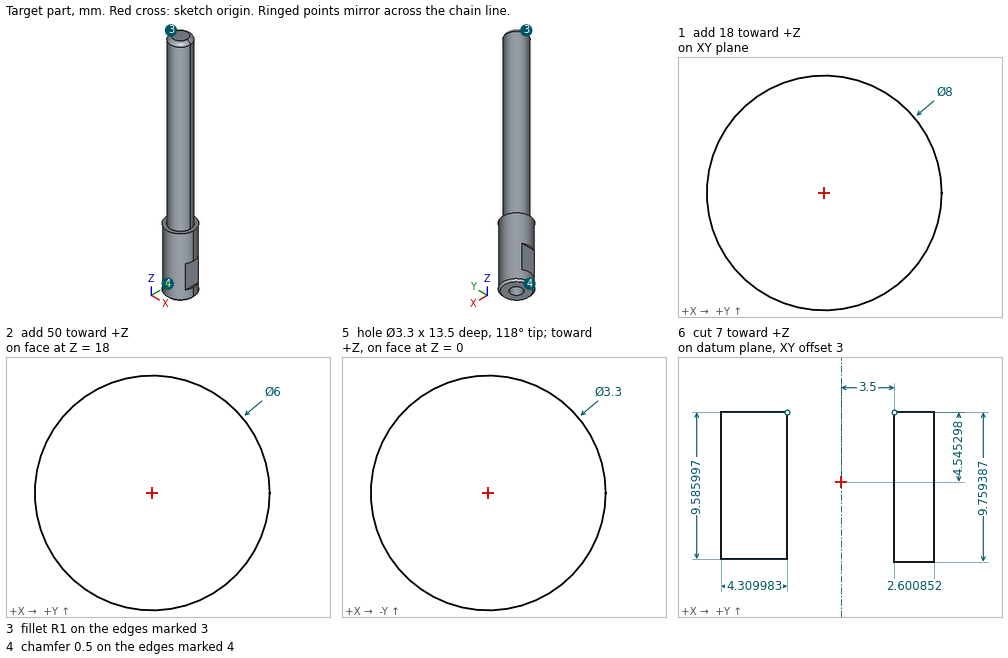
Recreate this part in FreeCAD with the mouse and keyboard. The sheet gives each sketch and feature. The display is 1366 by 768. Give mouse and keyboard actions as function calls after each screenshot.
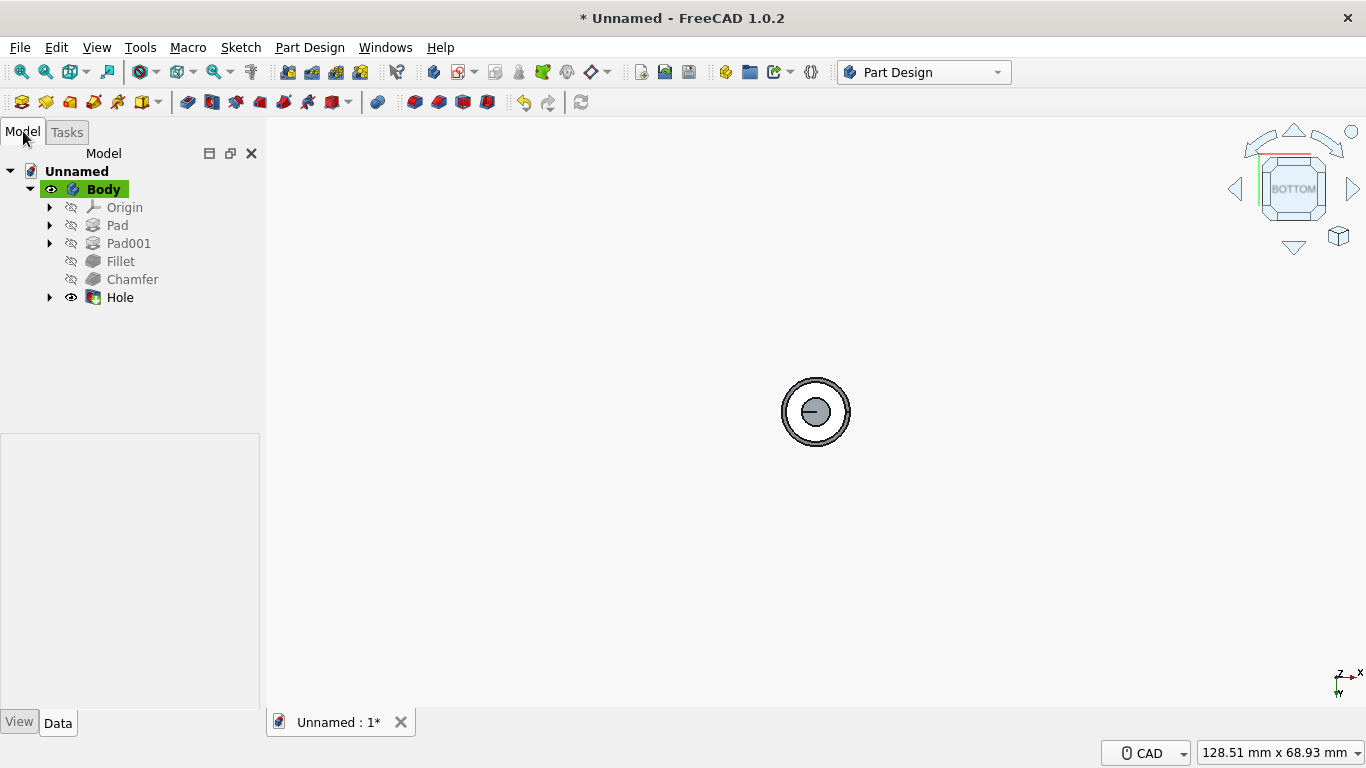
click(50, 207)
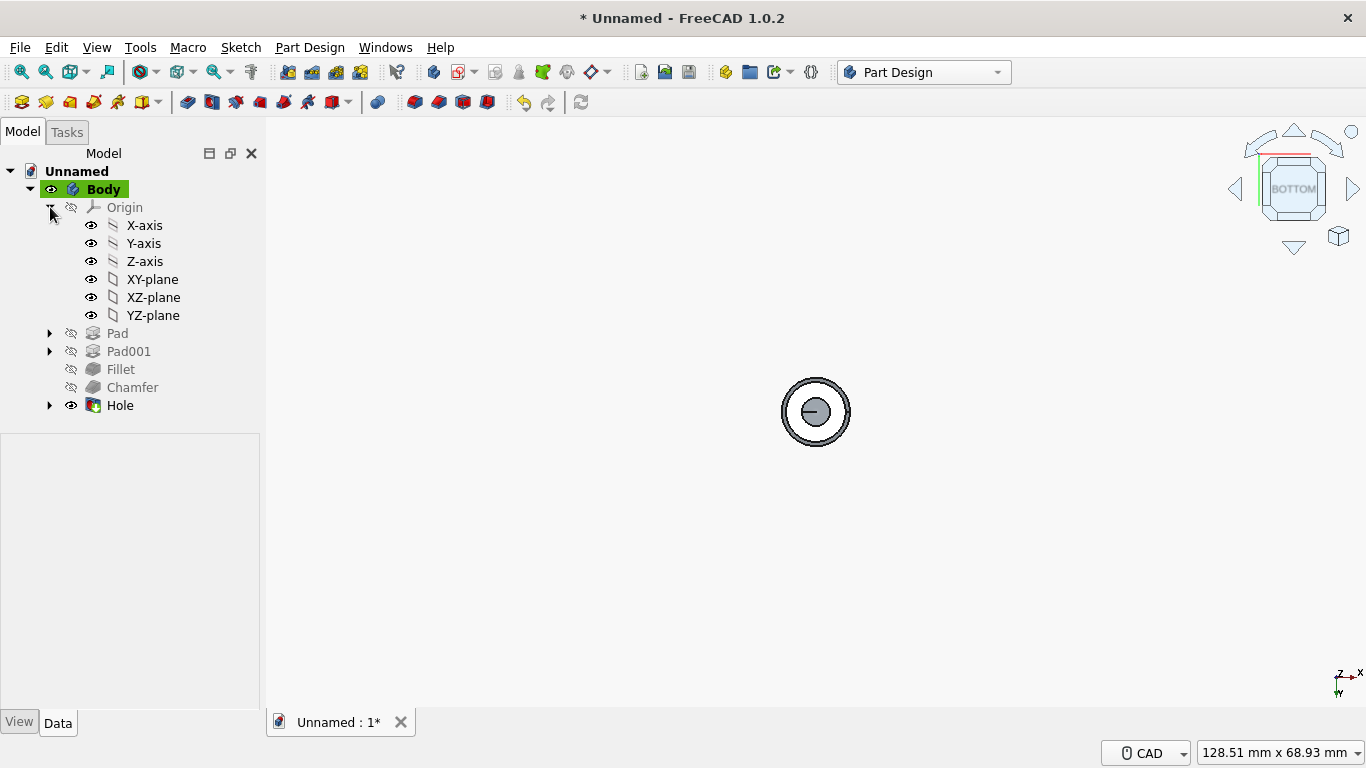
click(136, 279)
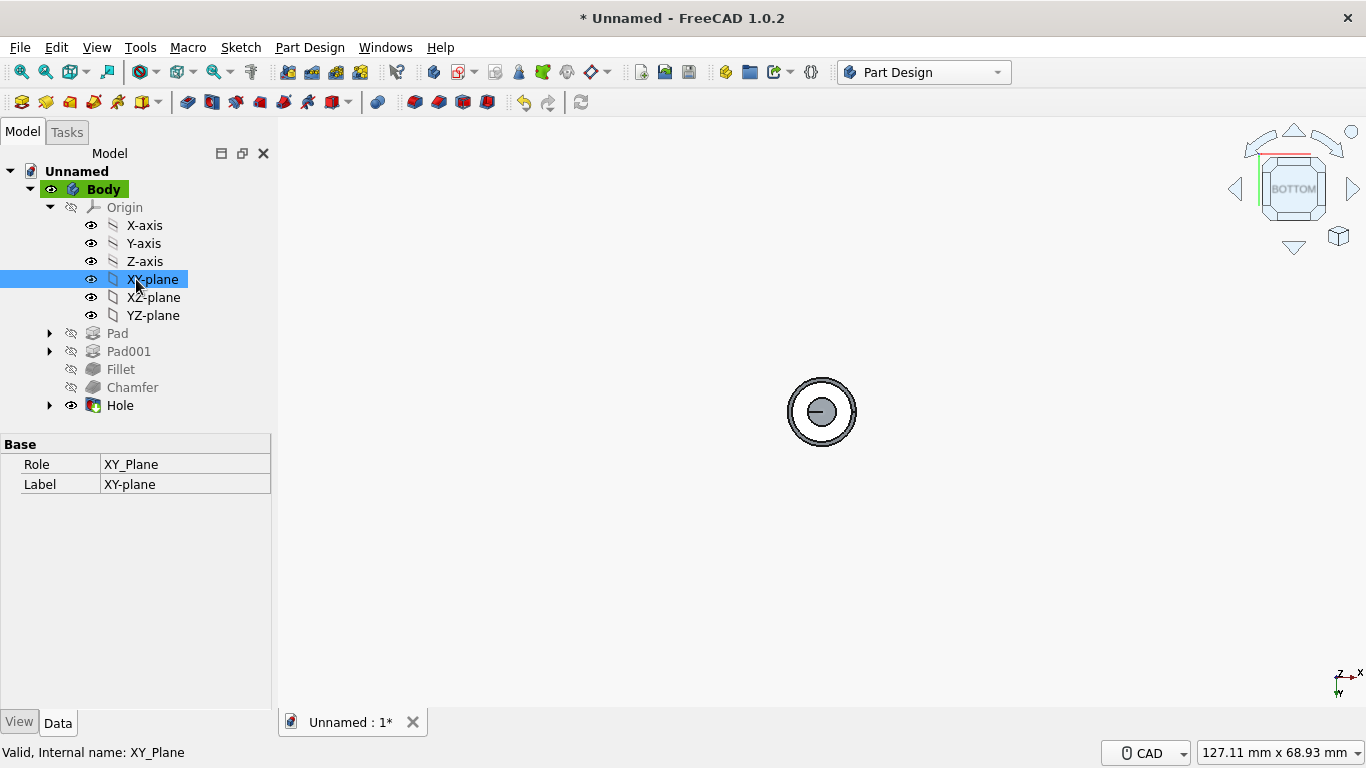
click(592, 72)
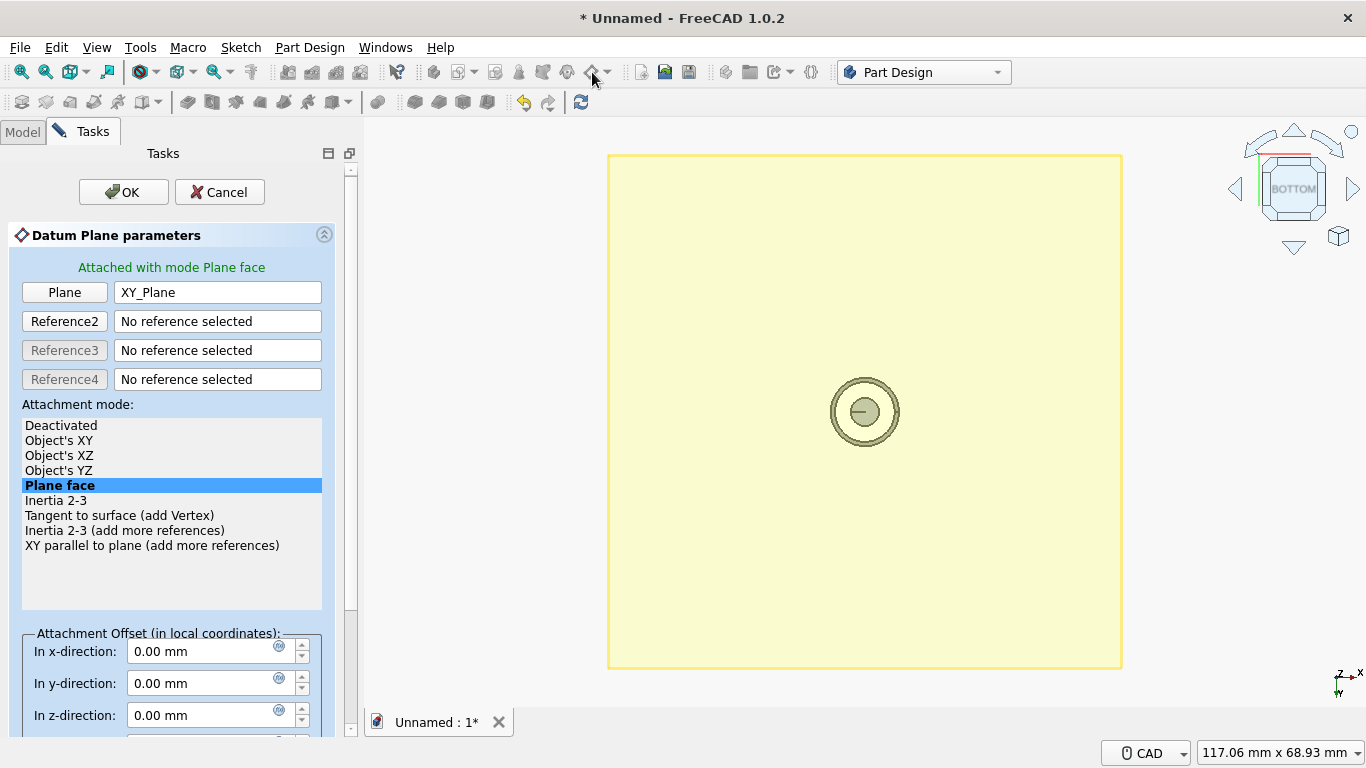
triple_click(210, 715)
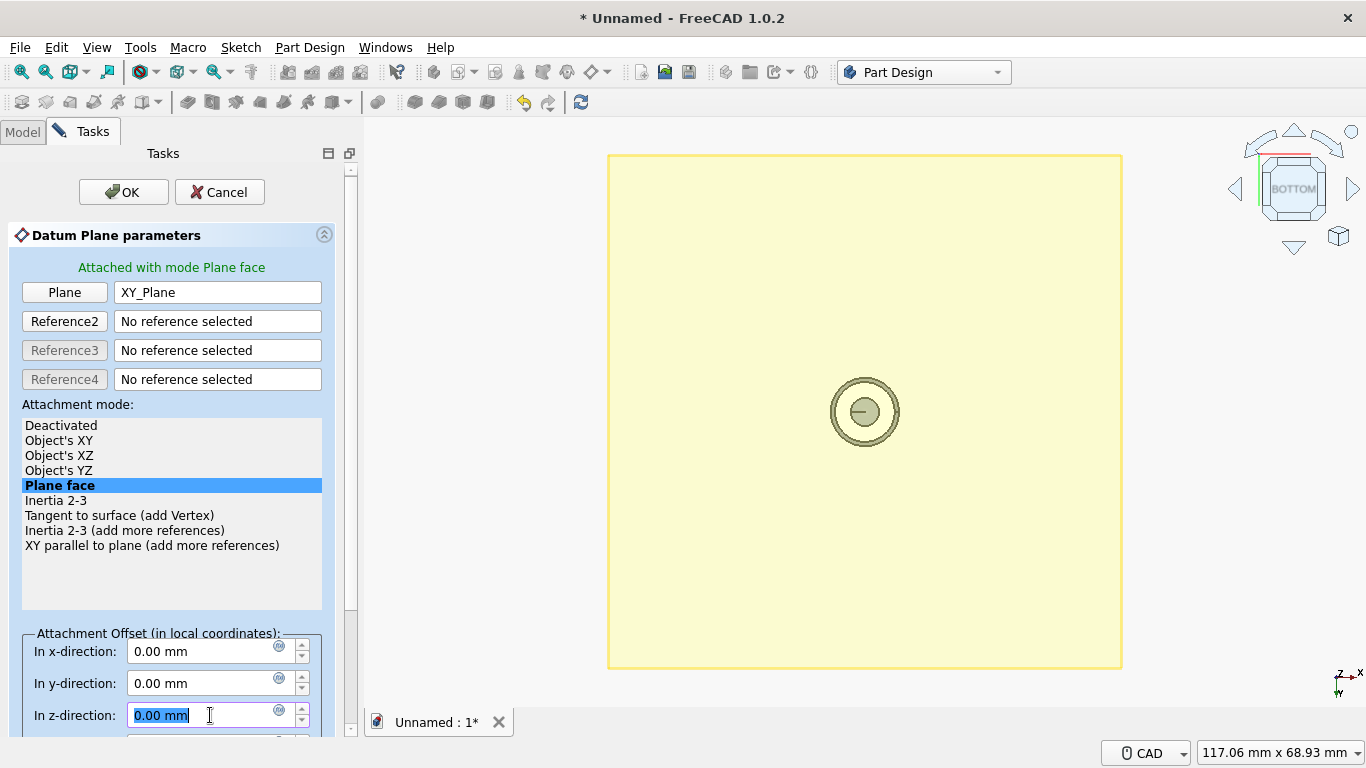
text(3)
key(Tab)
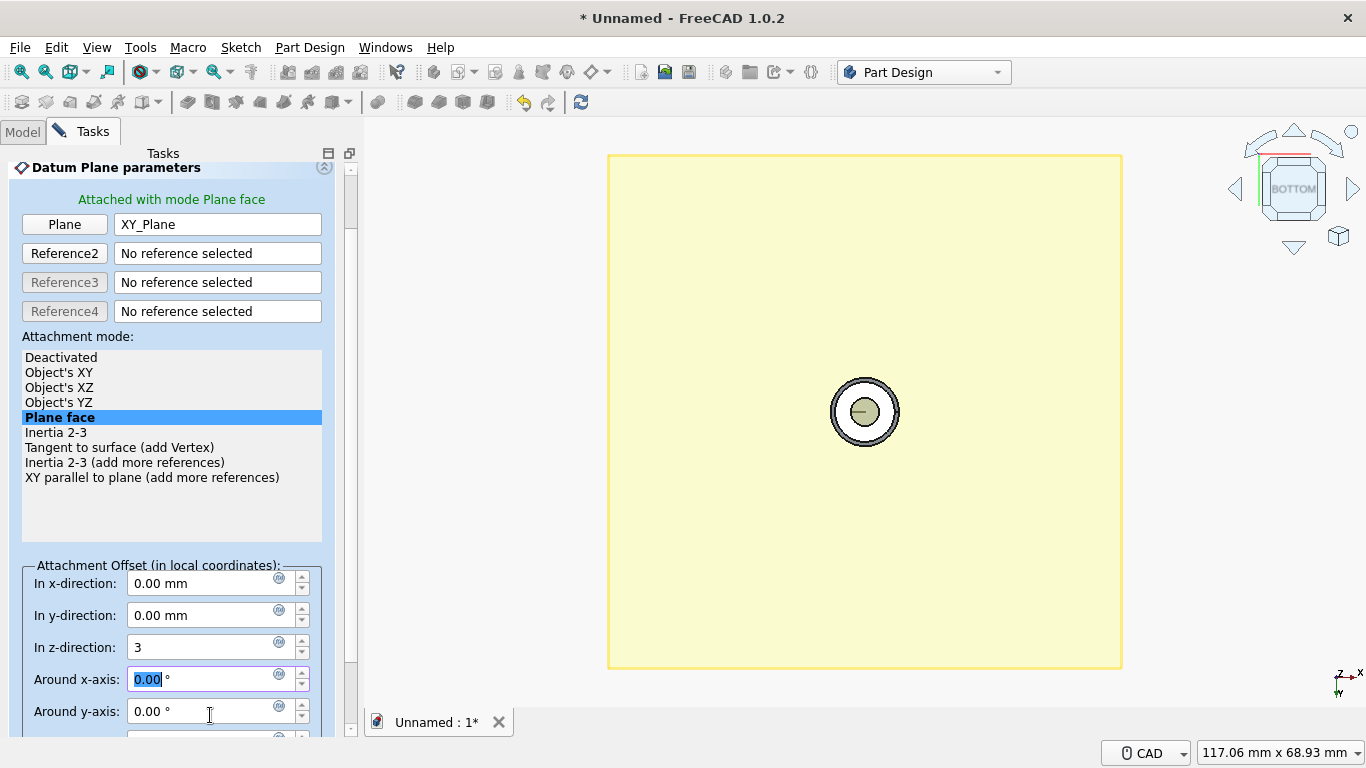
scroll(351, 450, up, 2)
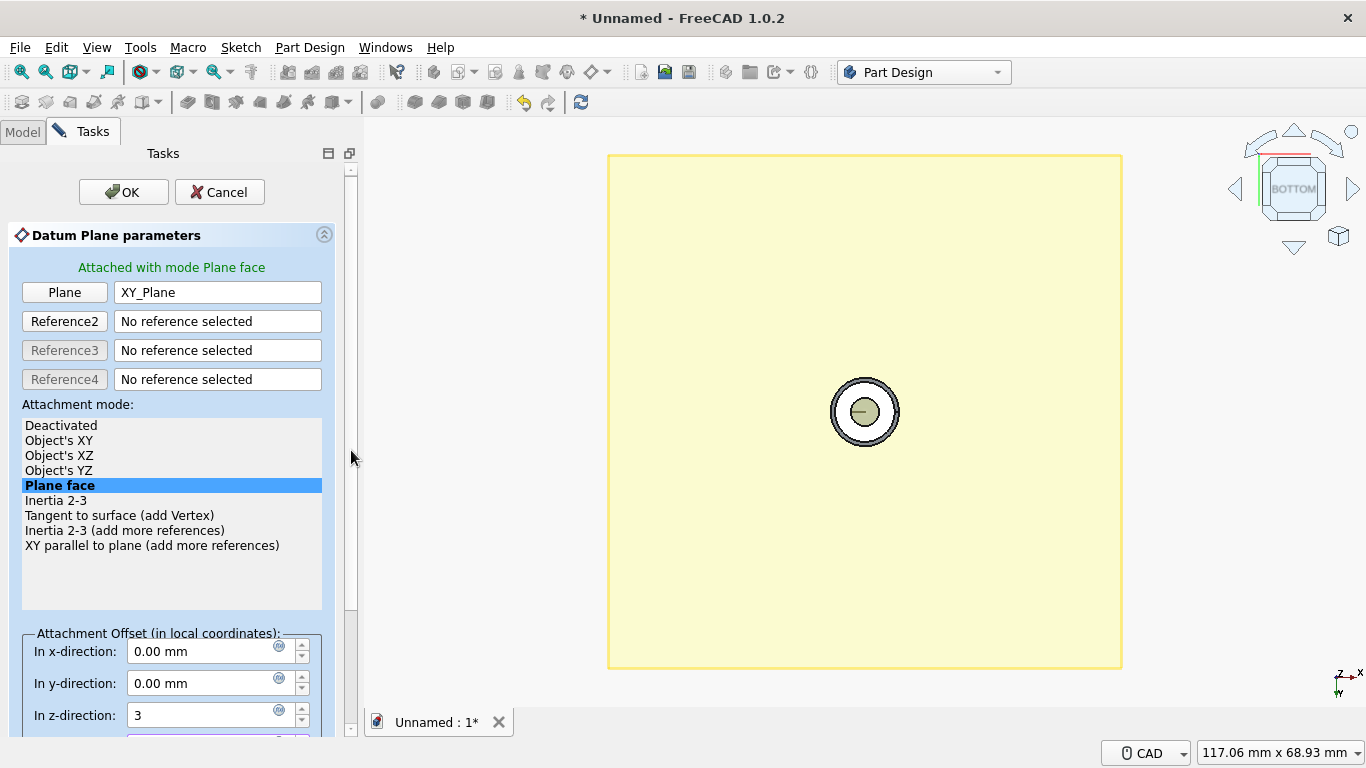
click(124, 192)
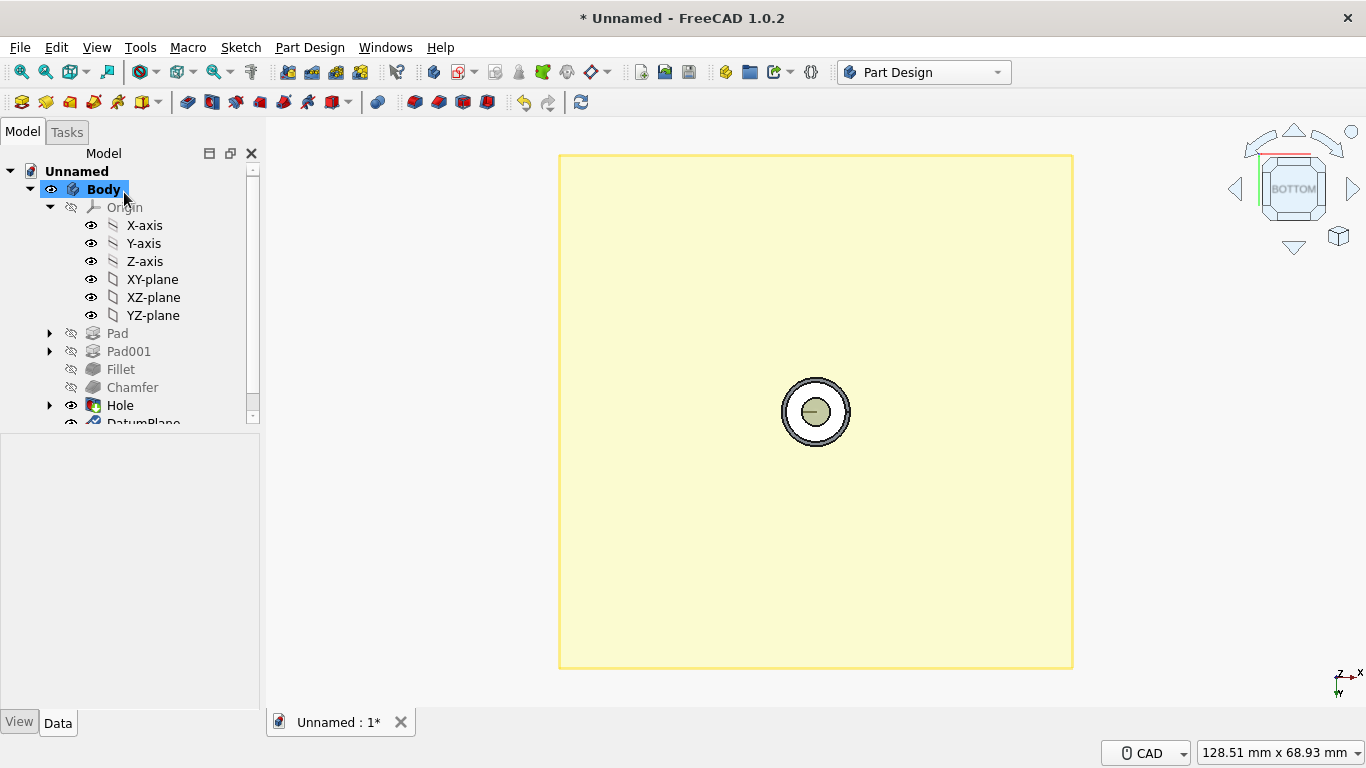
click(116, 423)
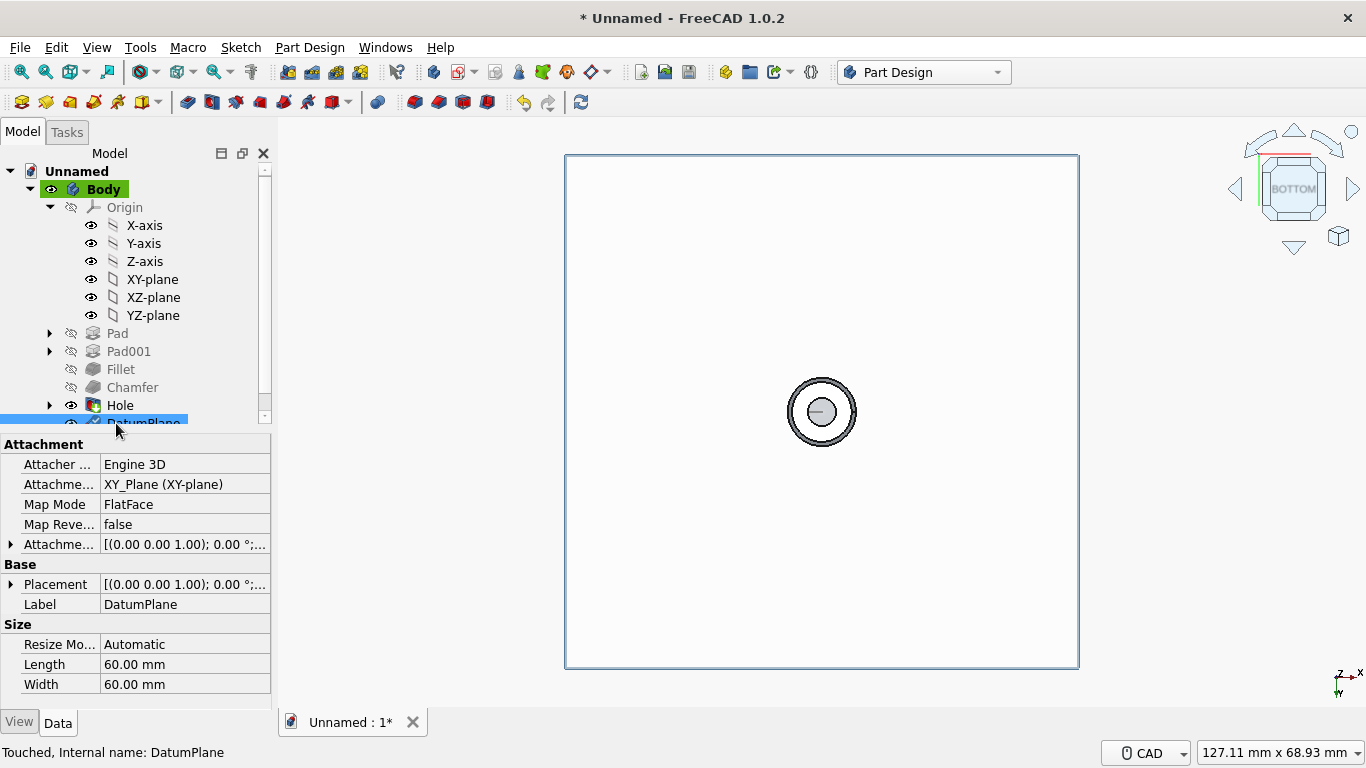
click(458, 72)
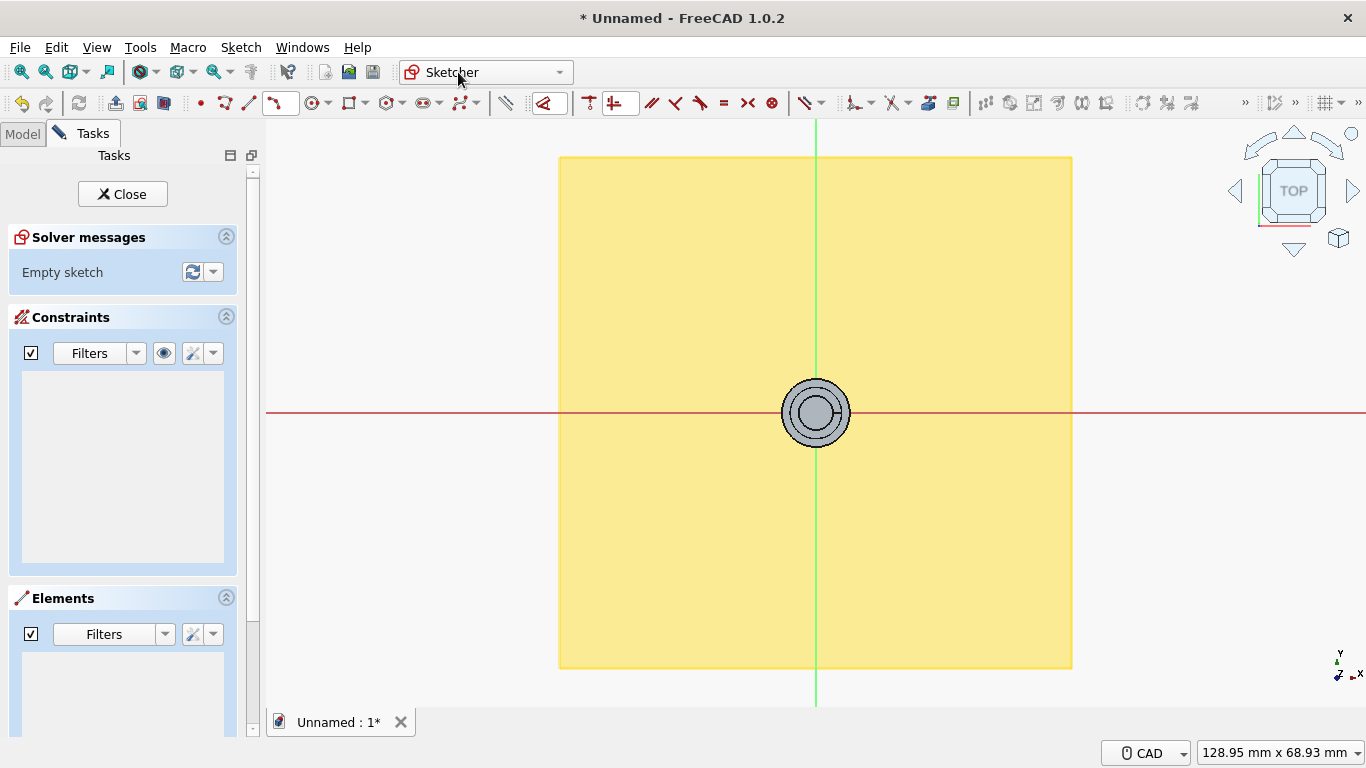
click(164, 104)